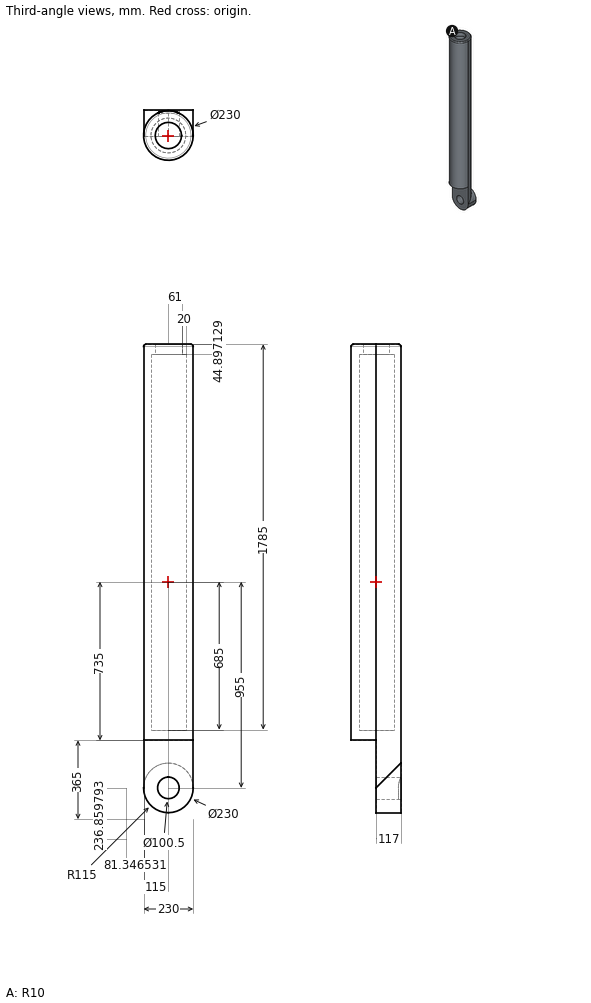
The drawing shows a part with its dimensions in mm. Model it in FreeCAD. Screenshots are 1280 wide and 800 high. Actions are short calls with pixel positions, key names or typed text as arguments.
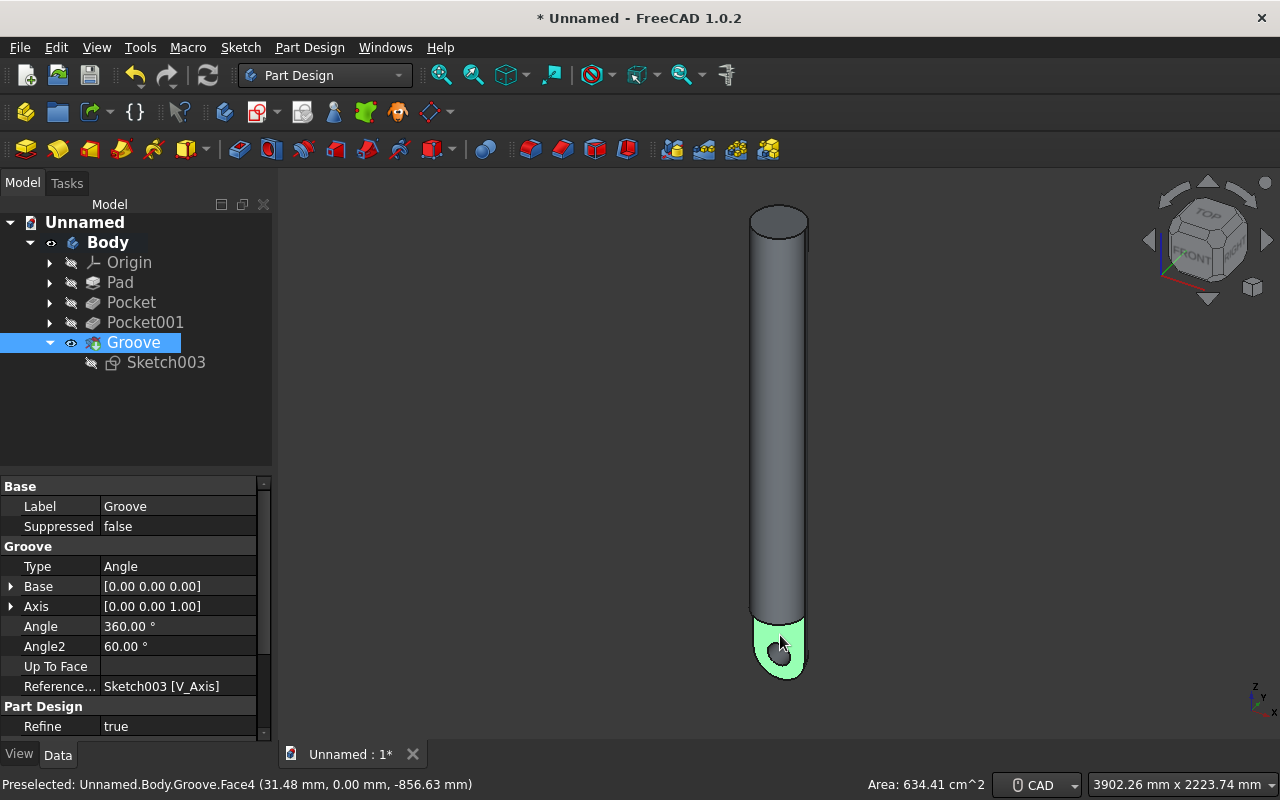
click(258, 112)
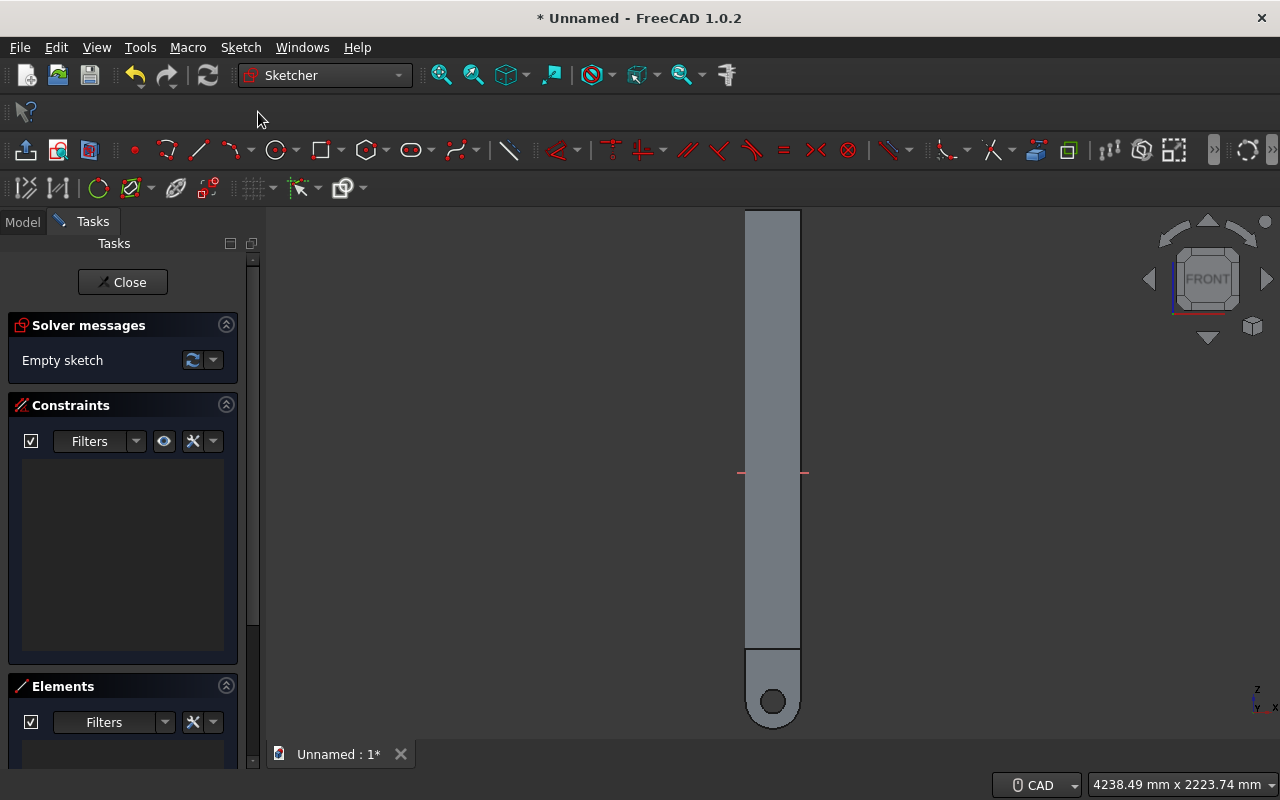
scroll(351, 697, down, 1)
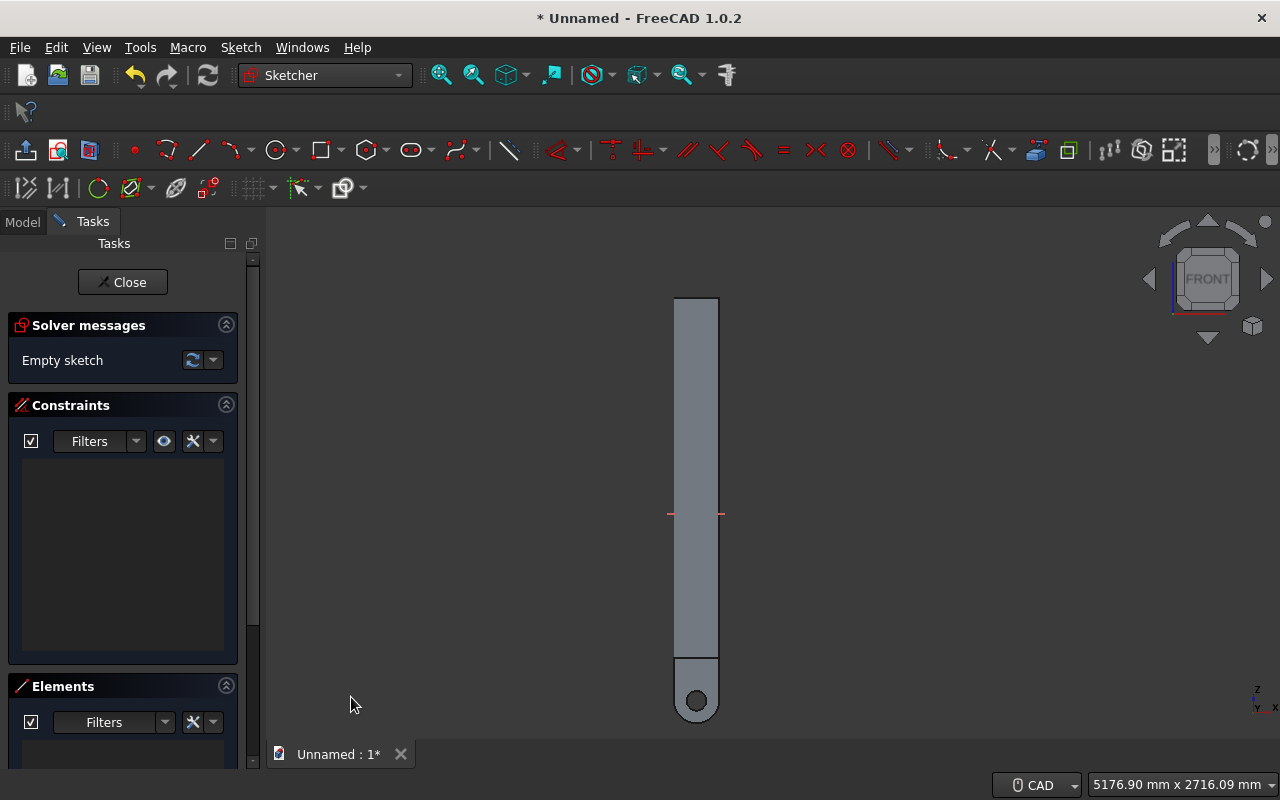
click(168, 150)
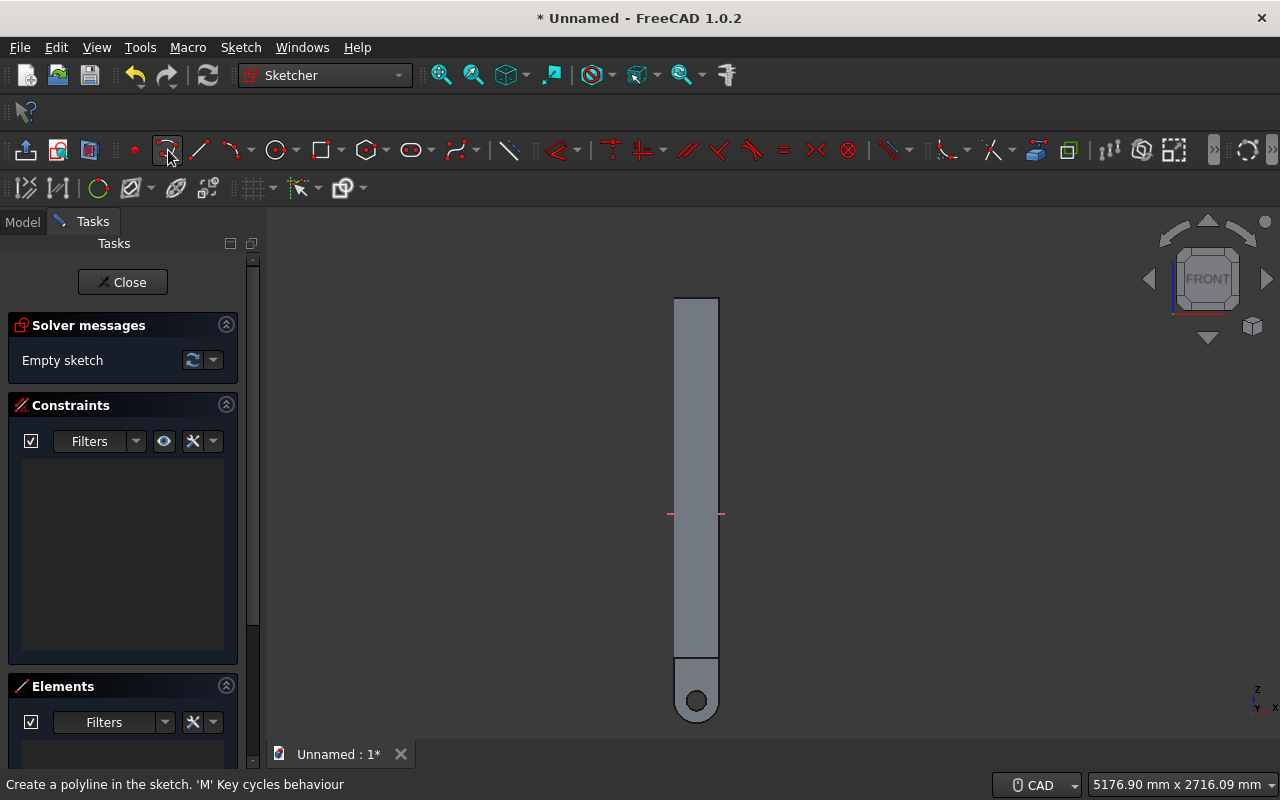
click(697, 648)
click(706, 298)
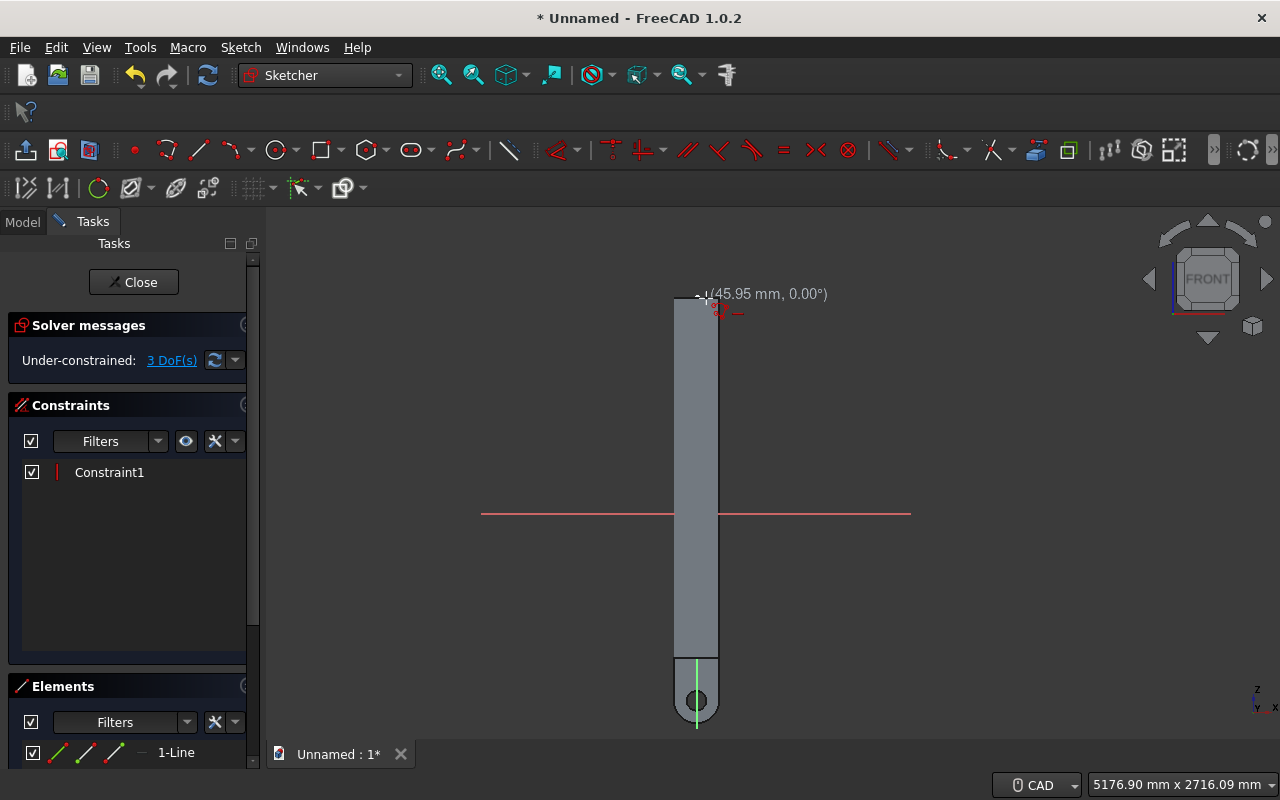
scroll(708, 298, up, 2)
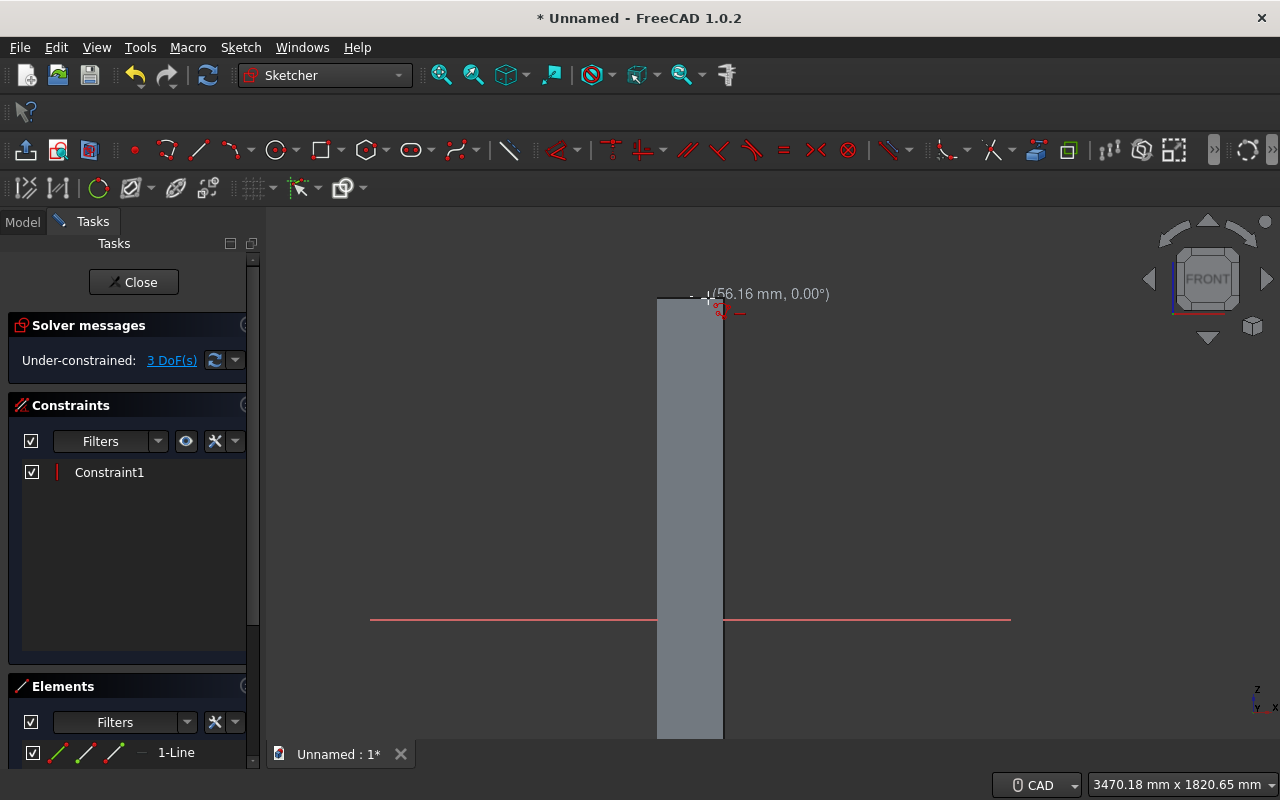
click(708, 298)
click(708, 312)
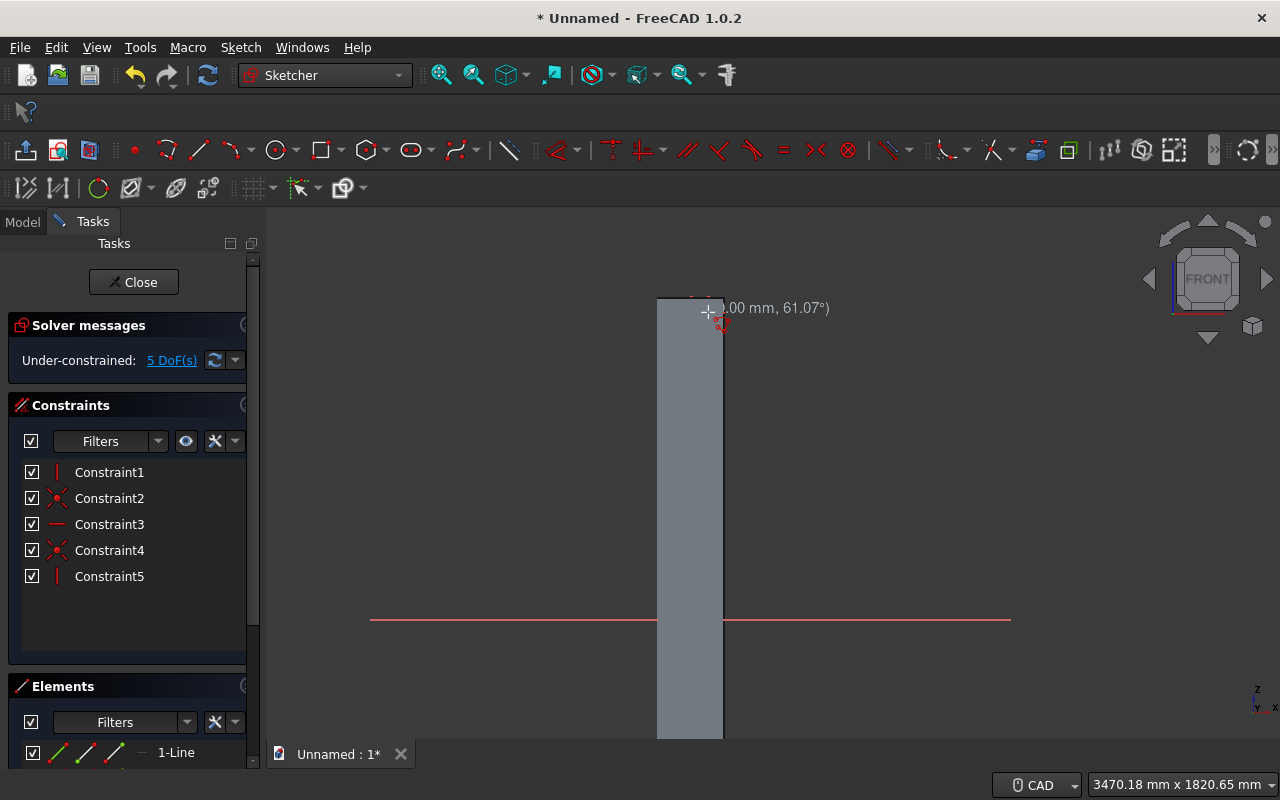
scroll(714, 312, up, 5)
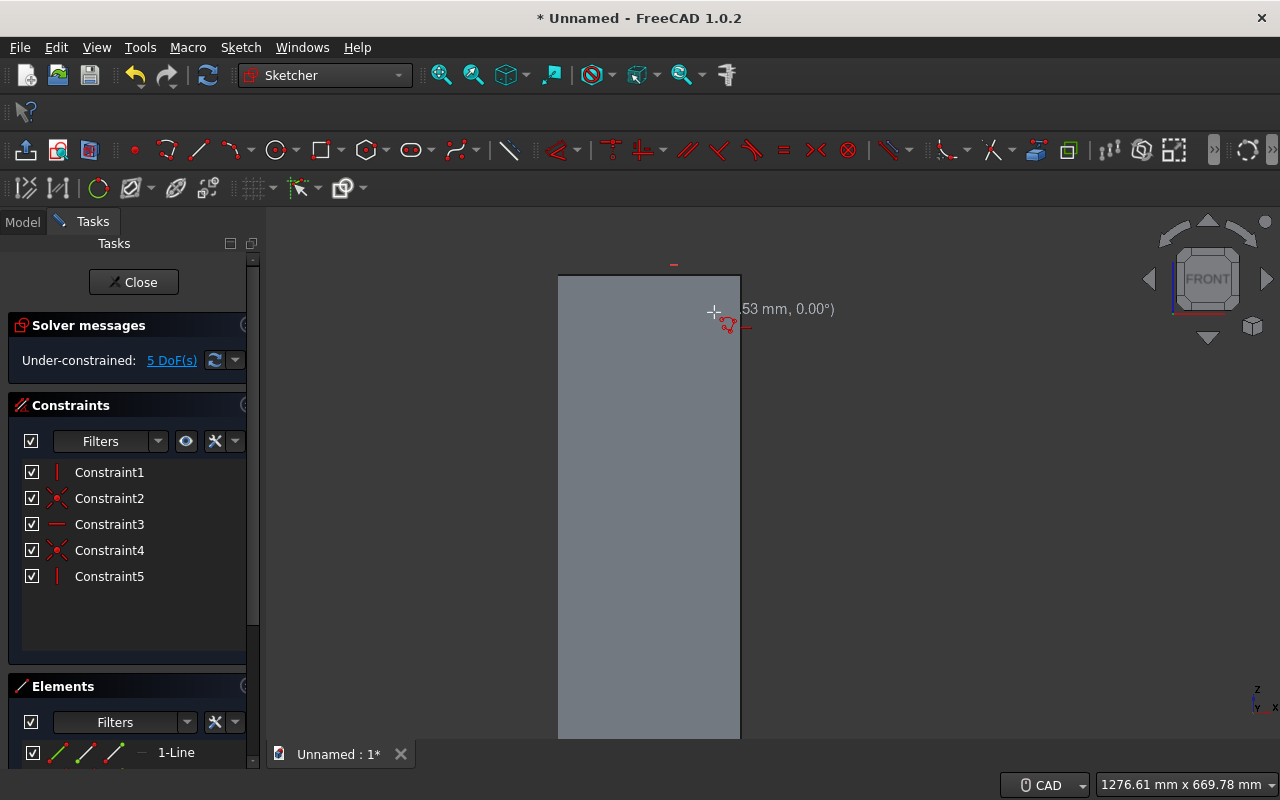
click(714, 312)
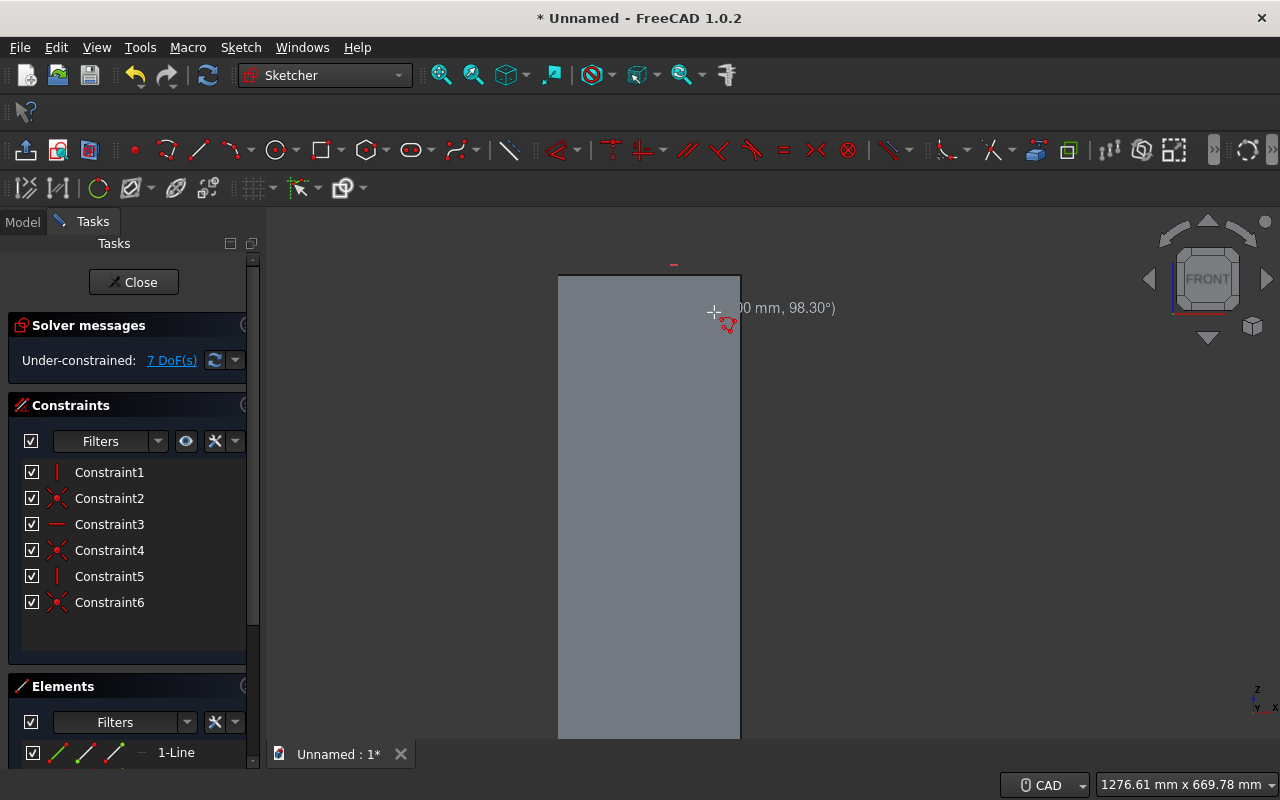
scroll(712, 306, down, 7)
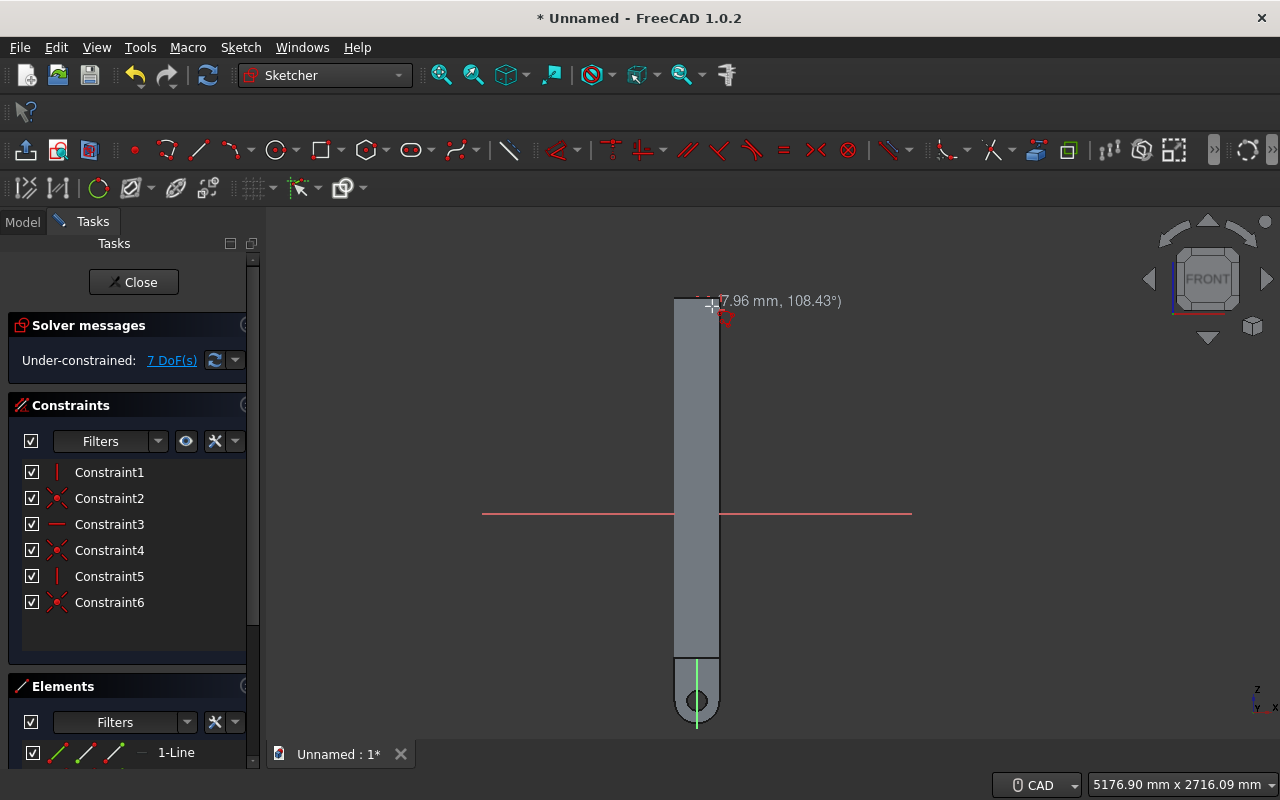
click(713, 648)
click(697, 649)
key(Escape)
key(Escape)